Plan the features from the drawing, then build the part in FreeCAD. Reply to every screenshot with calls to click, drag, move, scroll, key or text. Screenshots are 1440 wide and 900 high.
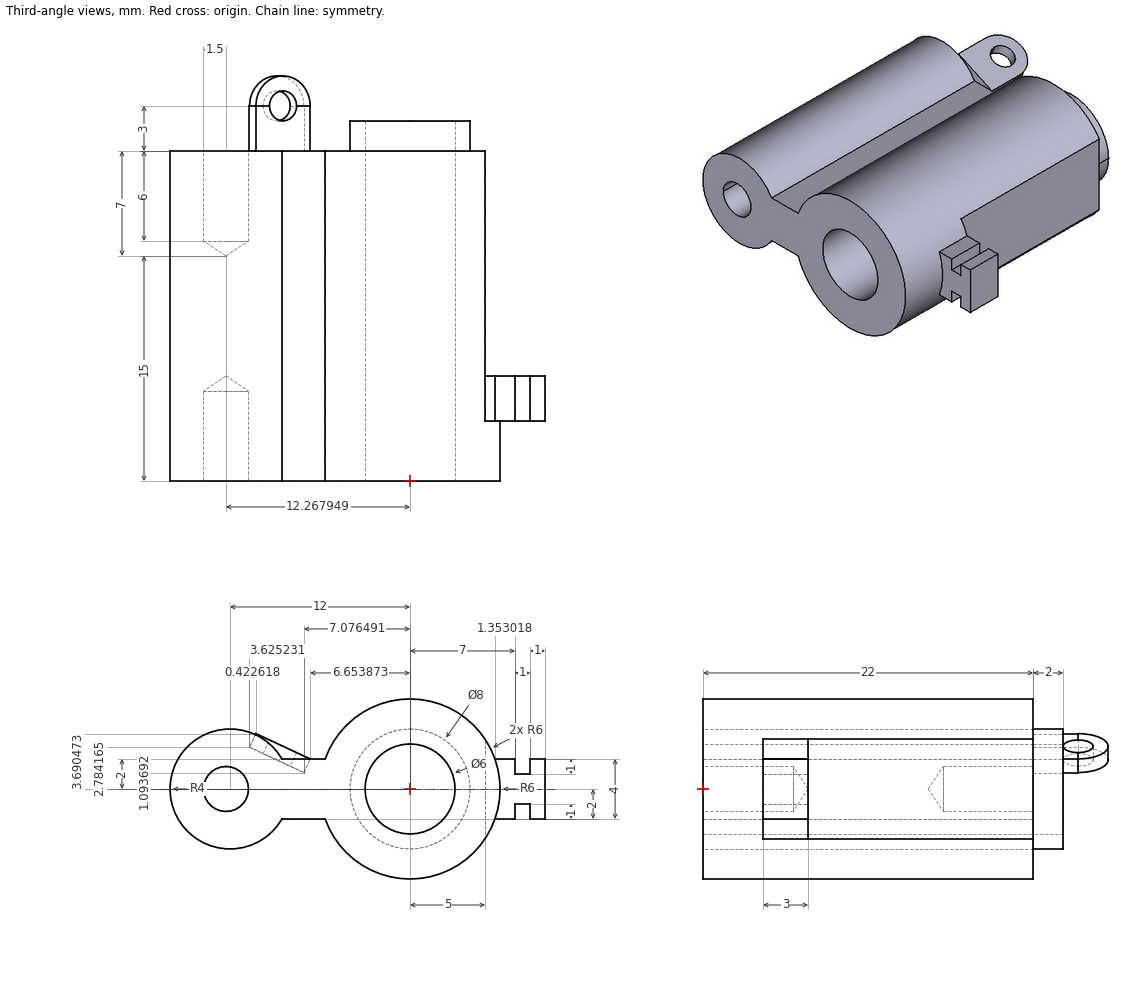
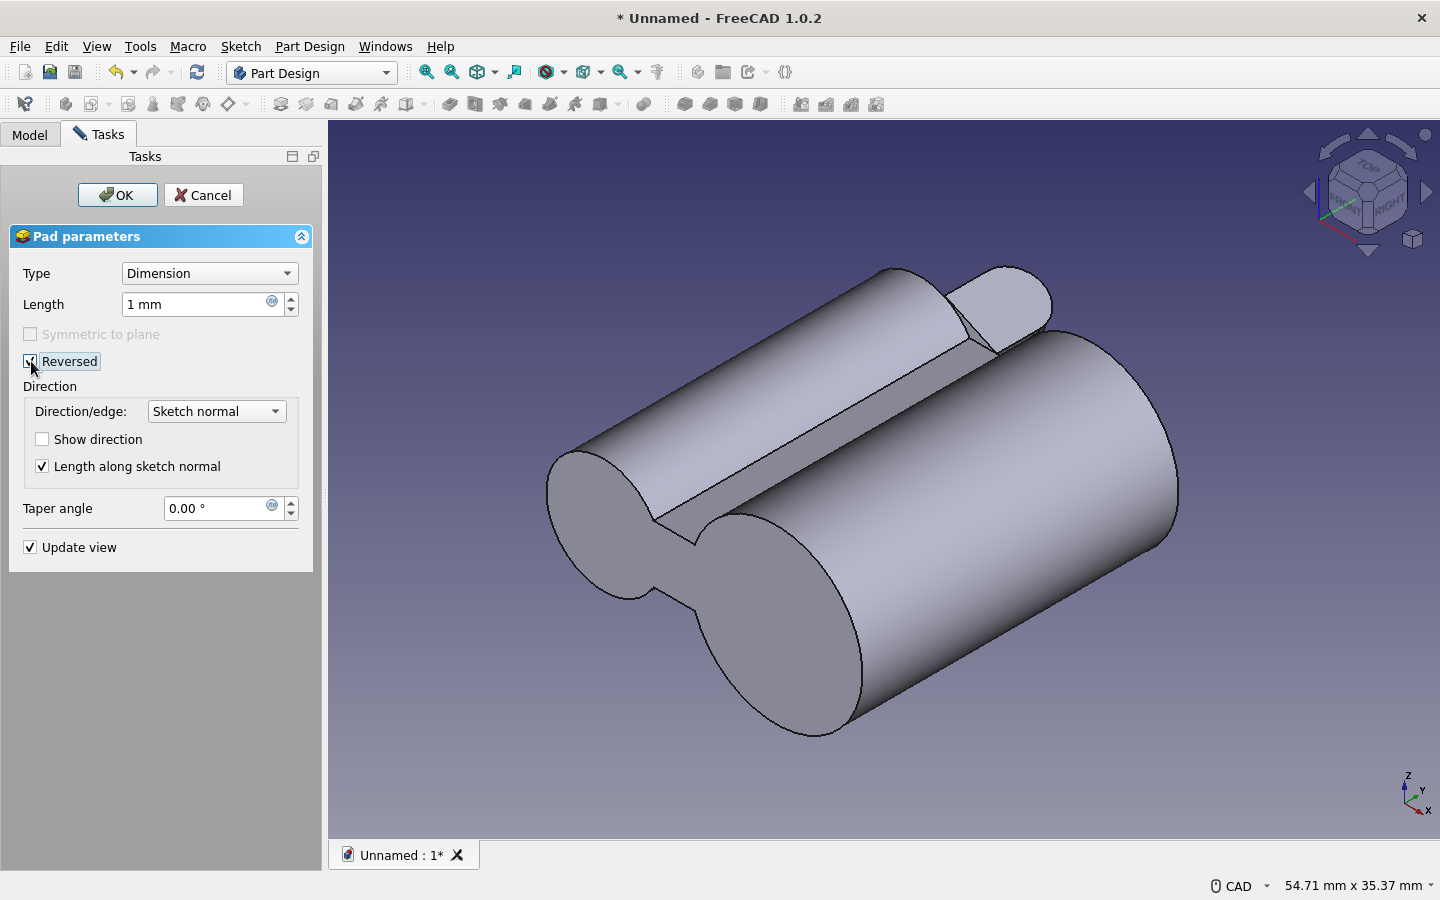
click(118, 195)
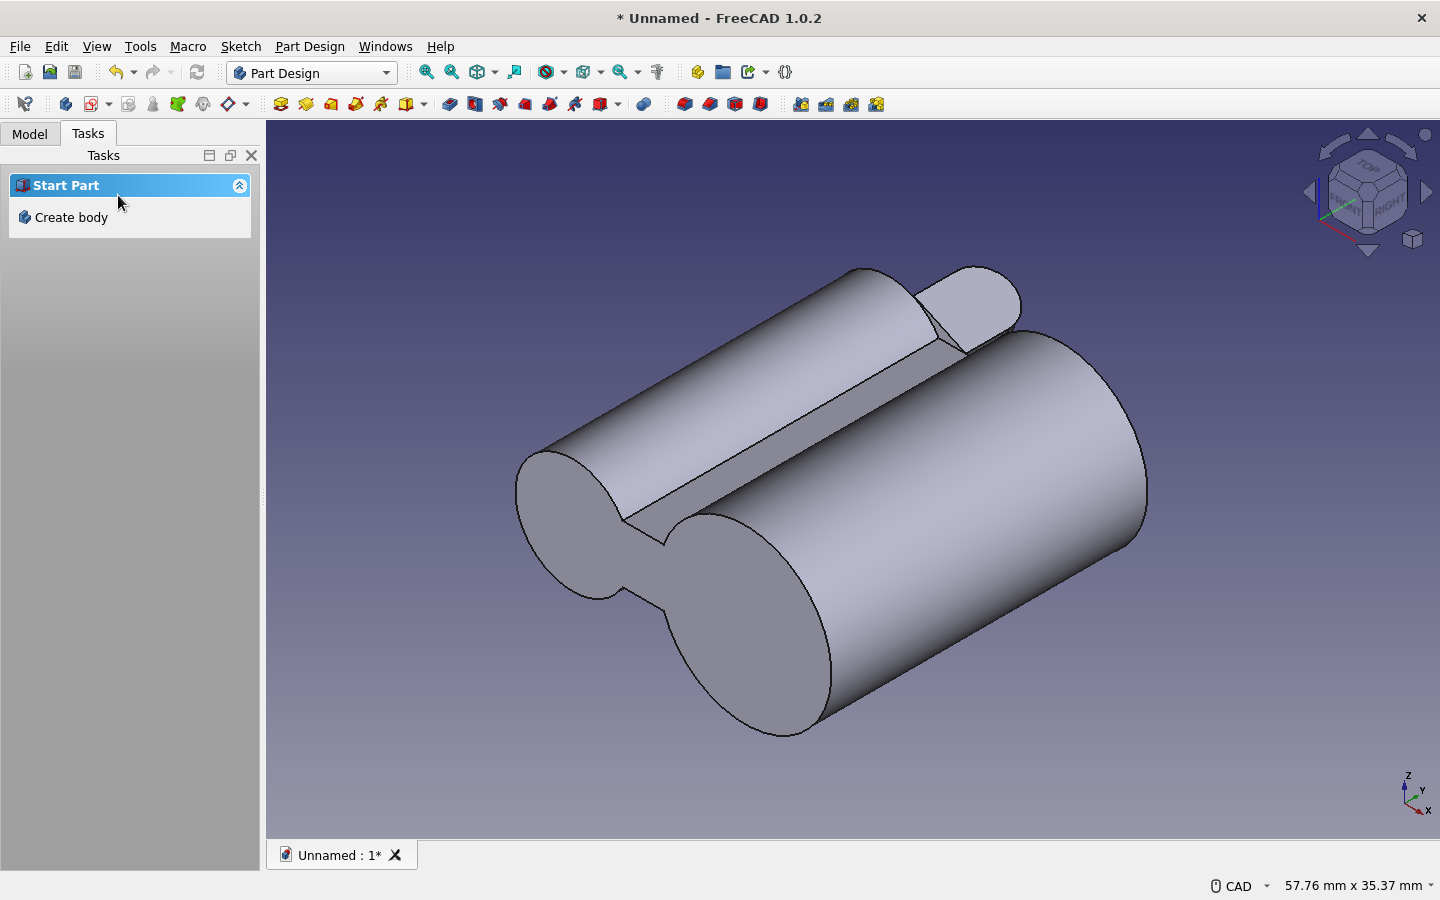
click(976, 303)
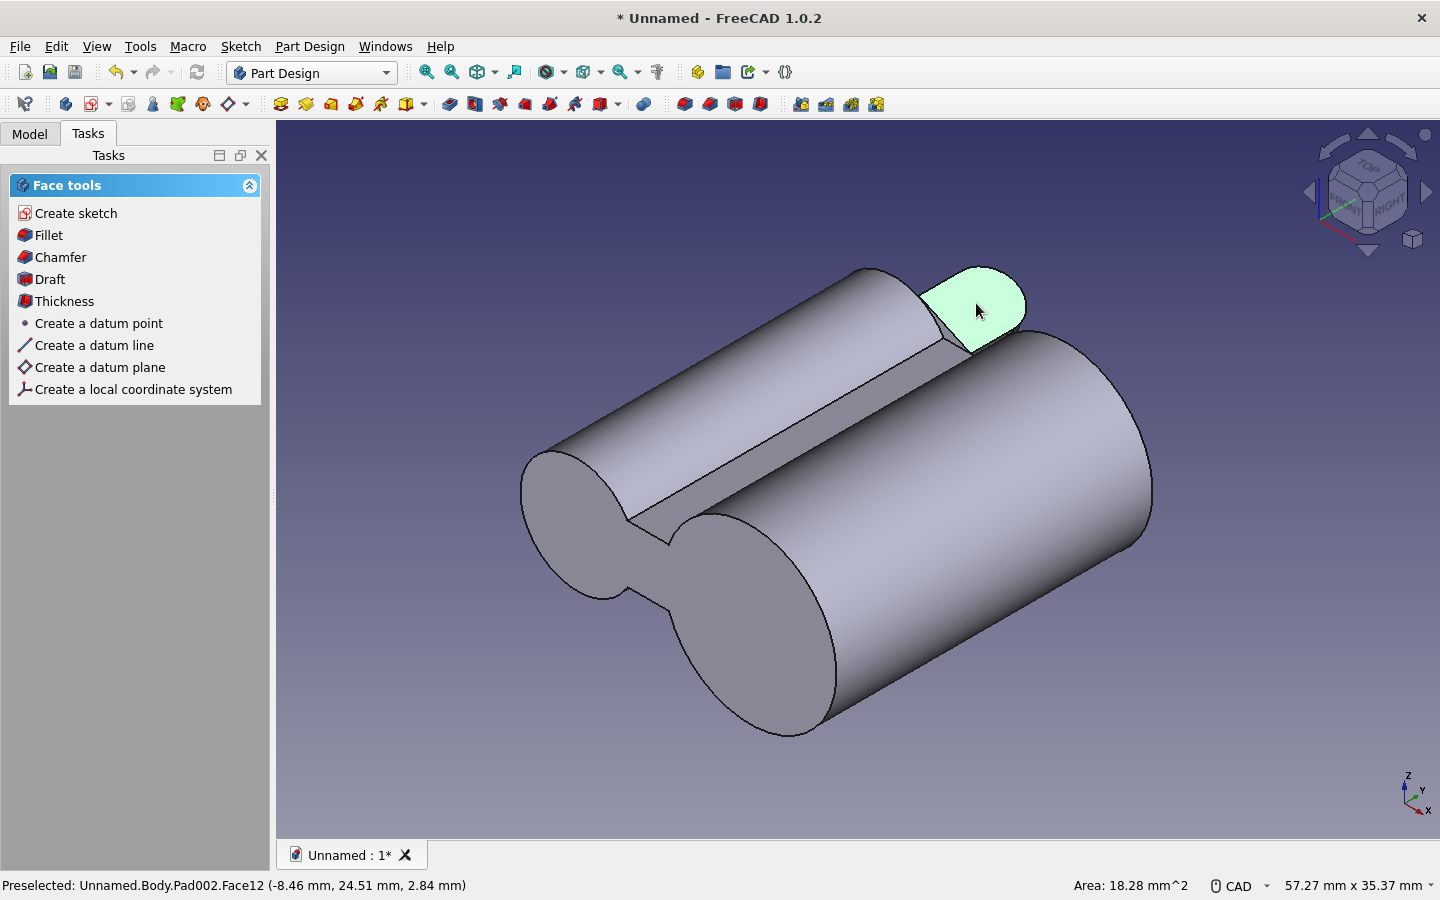
click(90, 104)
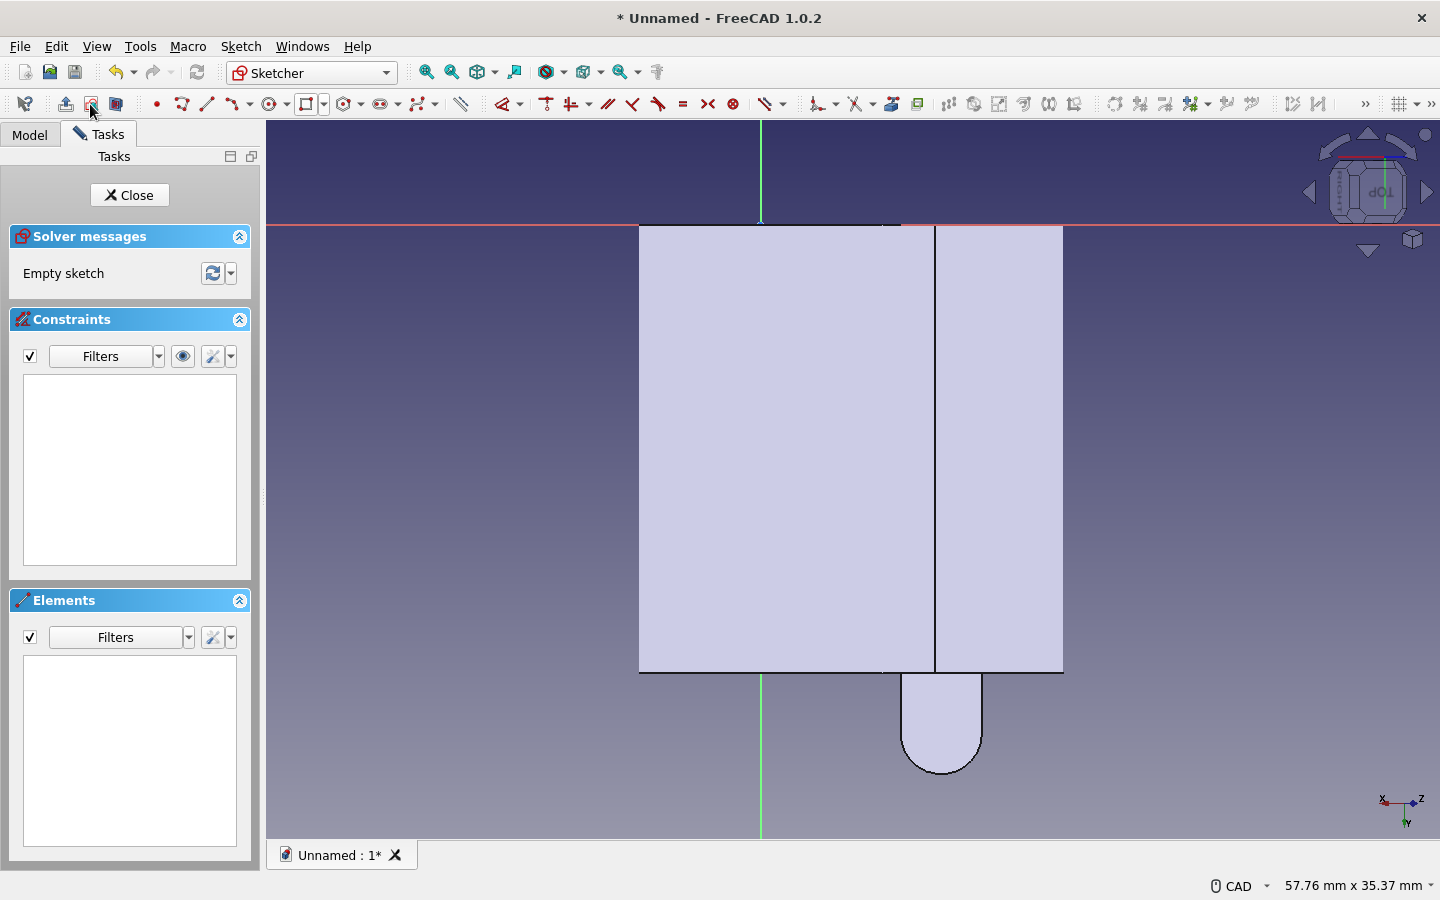
click(116, 104)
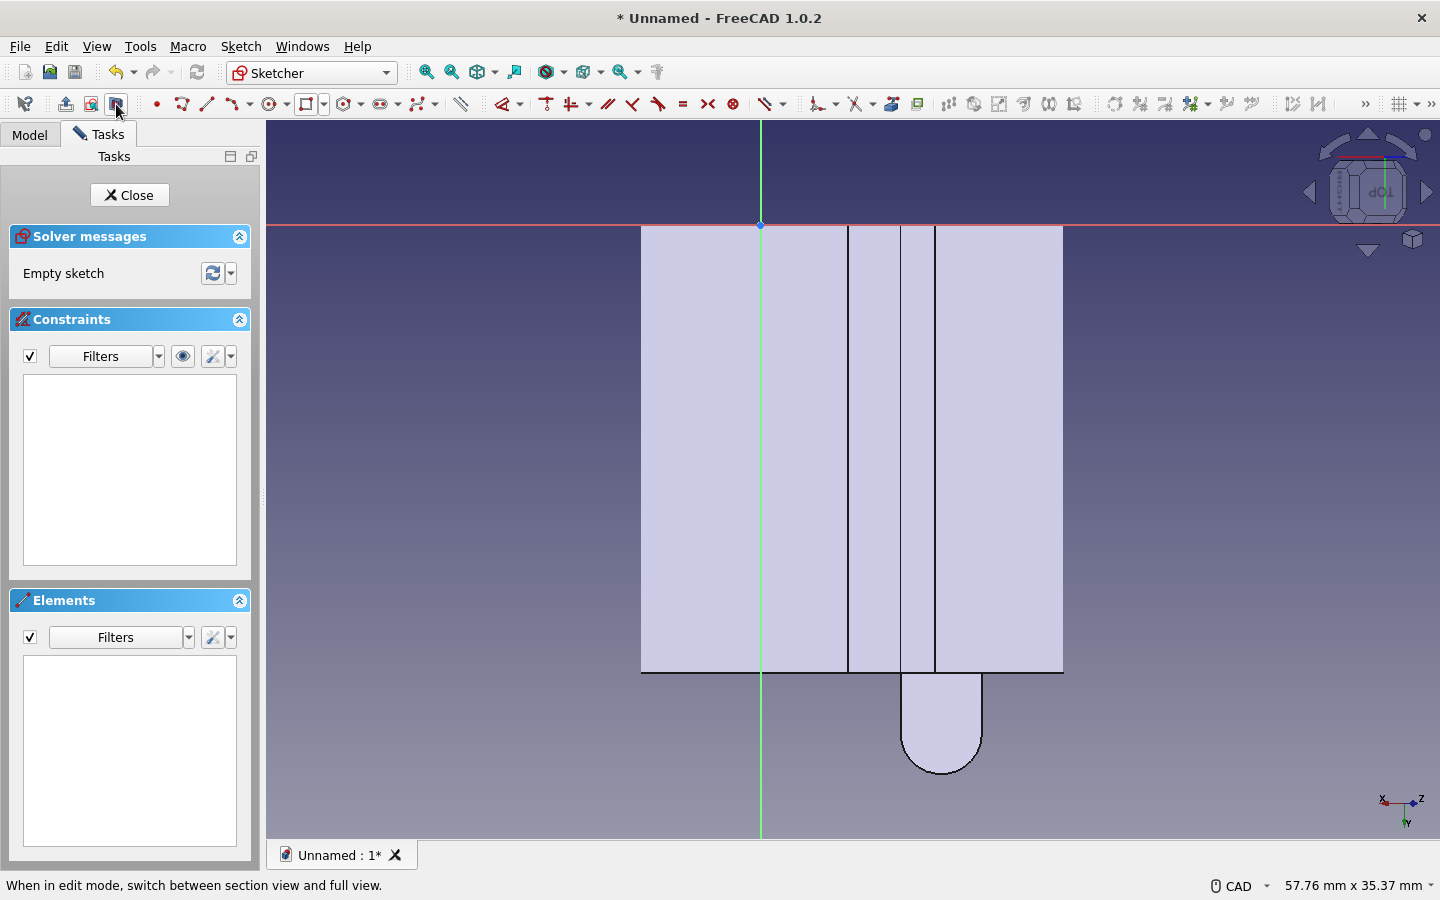
scroll(957, 759, up, 12)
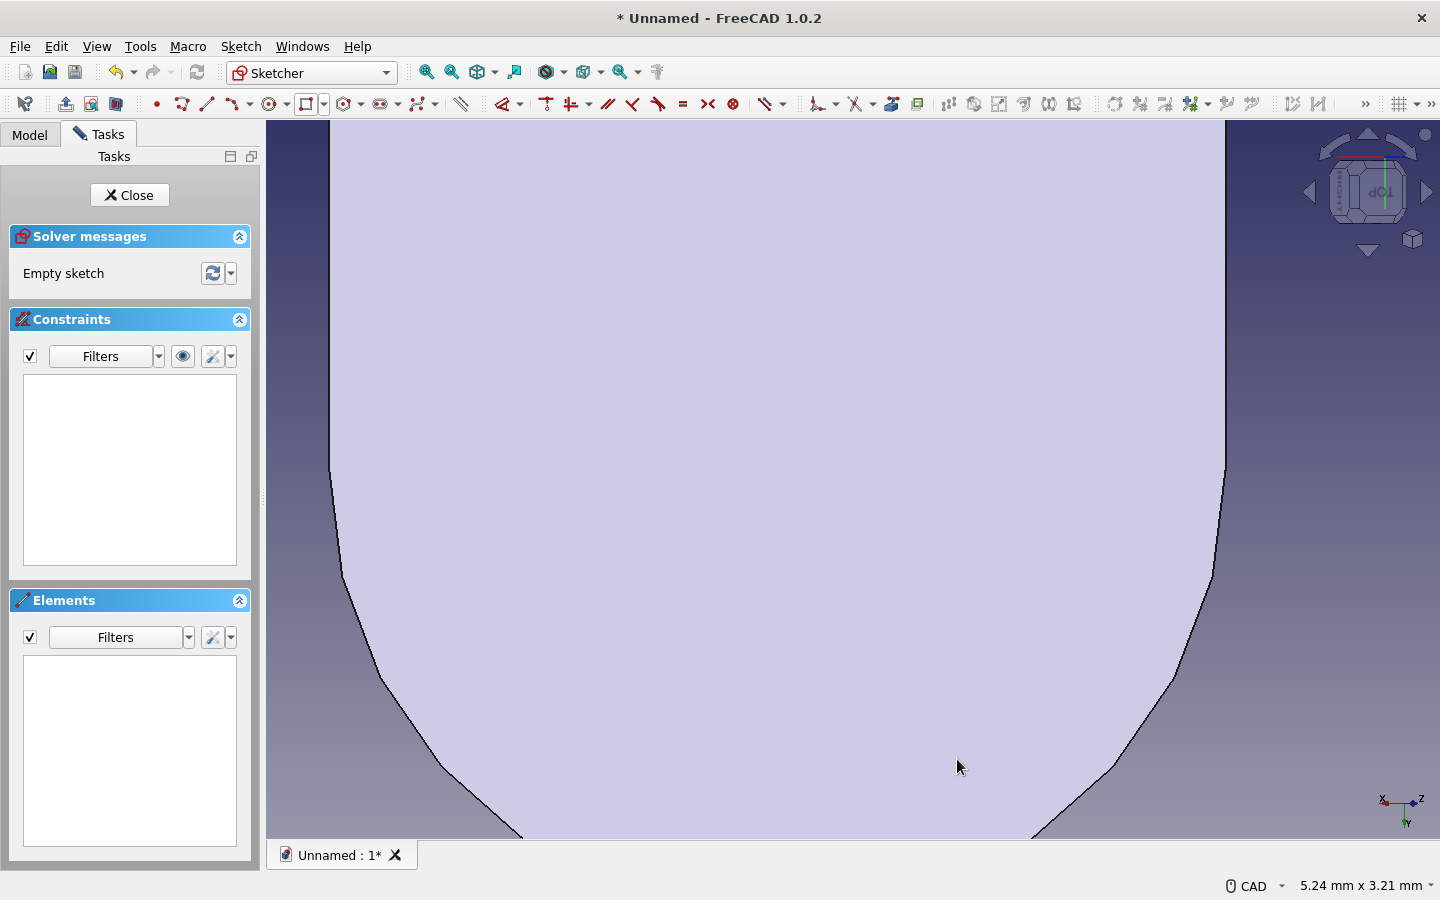
click(268, 104)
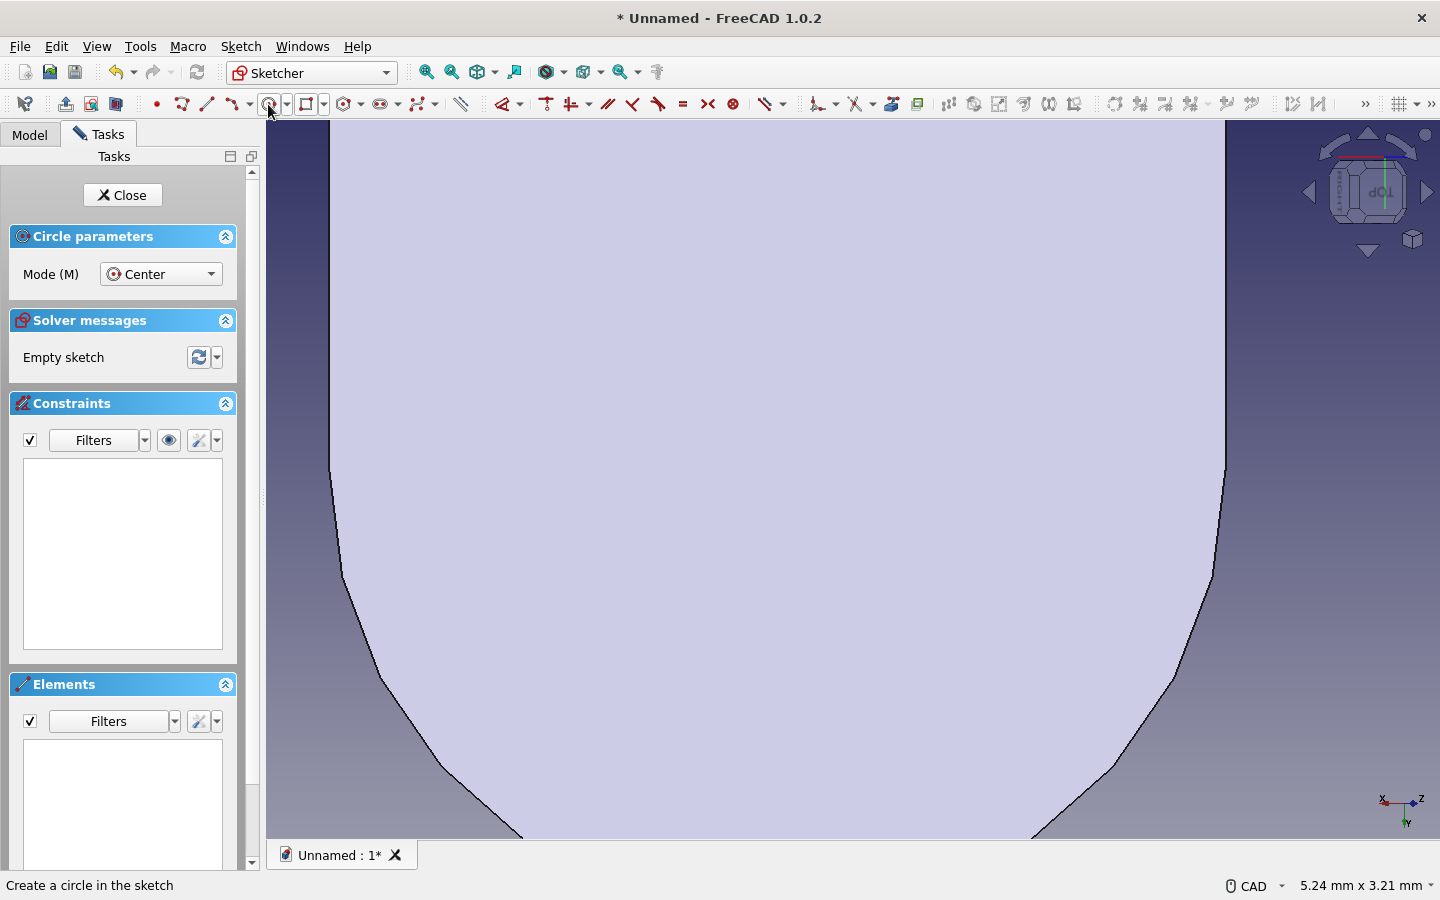
click(777, 470)
move(936, 311)